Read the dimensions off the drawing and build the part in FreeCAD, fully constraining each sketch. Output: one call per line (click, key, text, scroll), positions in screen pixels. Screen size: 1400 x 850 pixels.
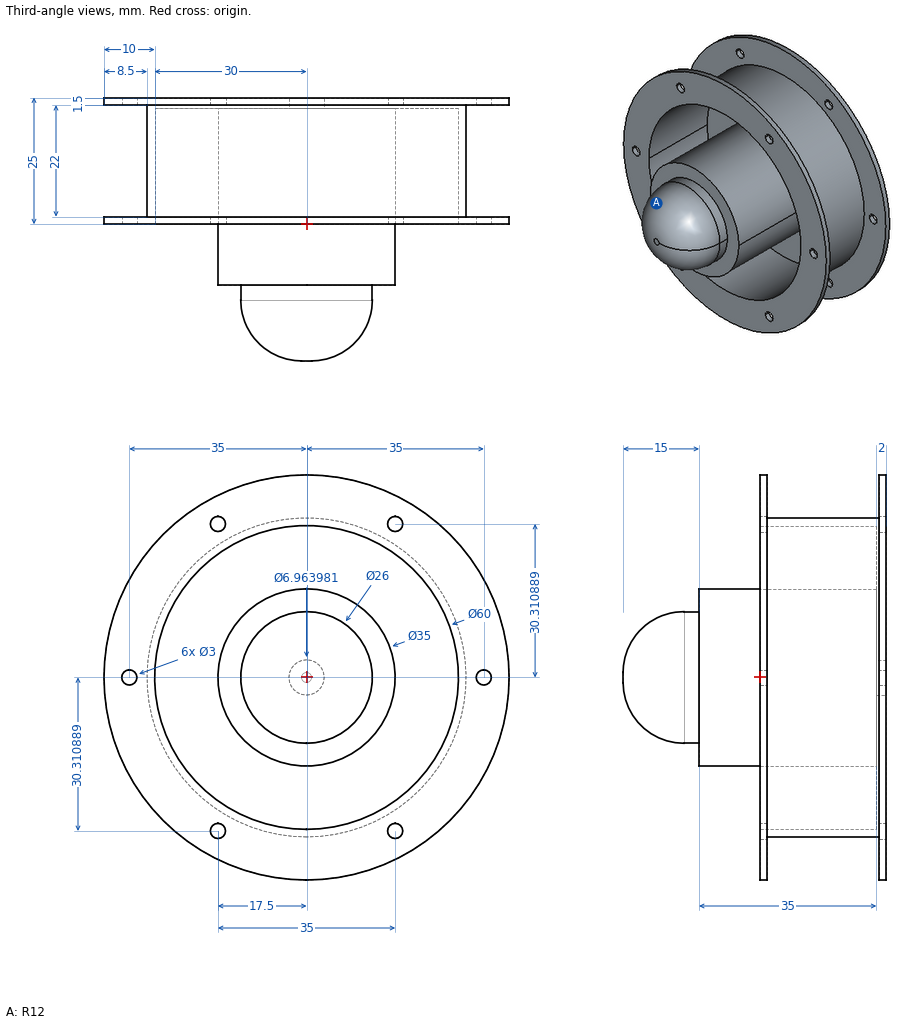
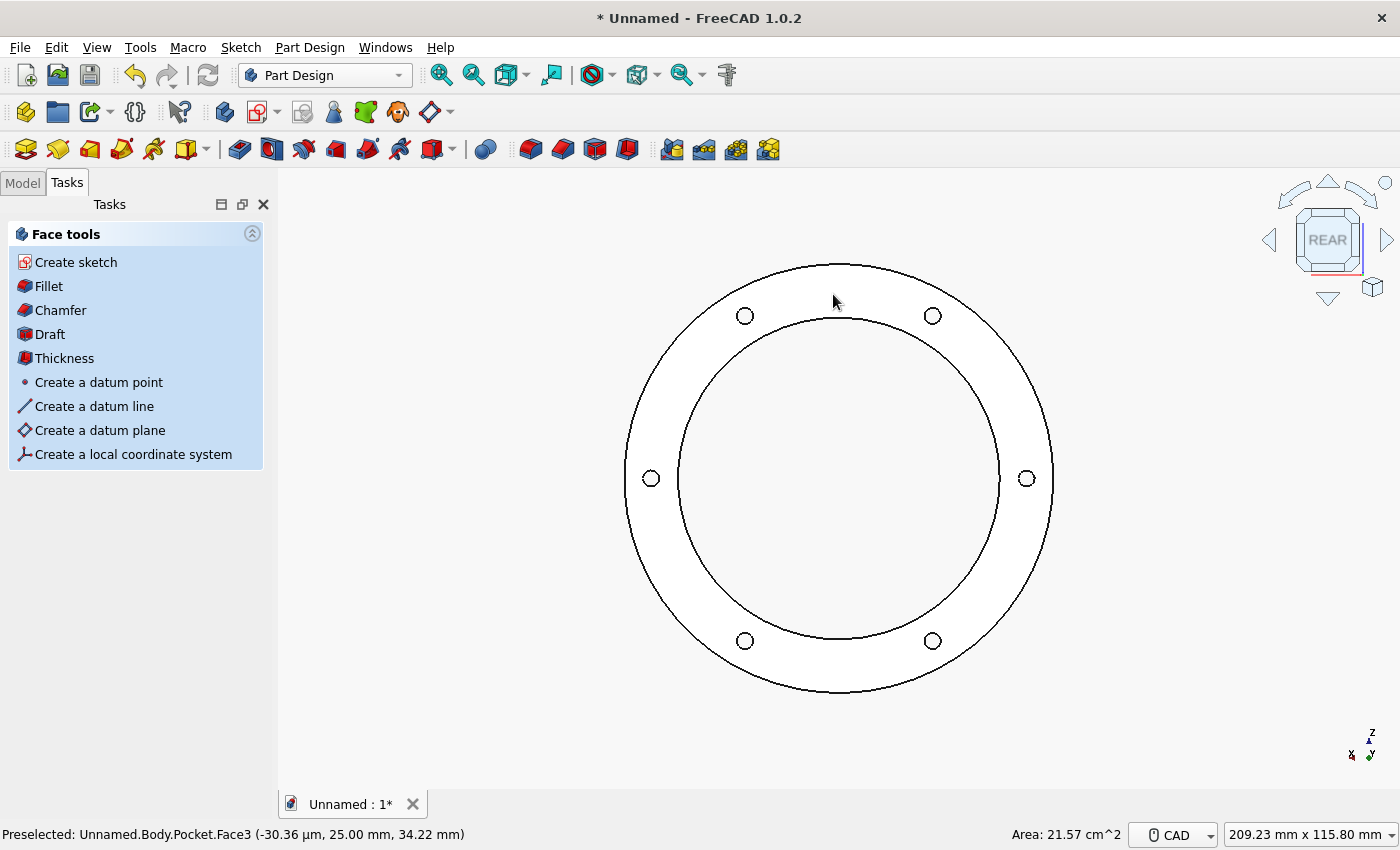
click(258, 112)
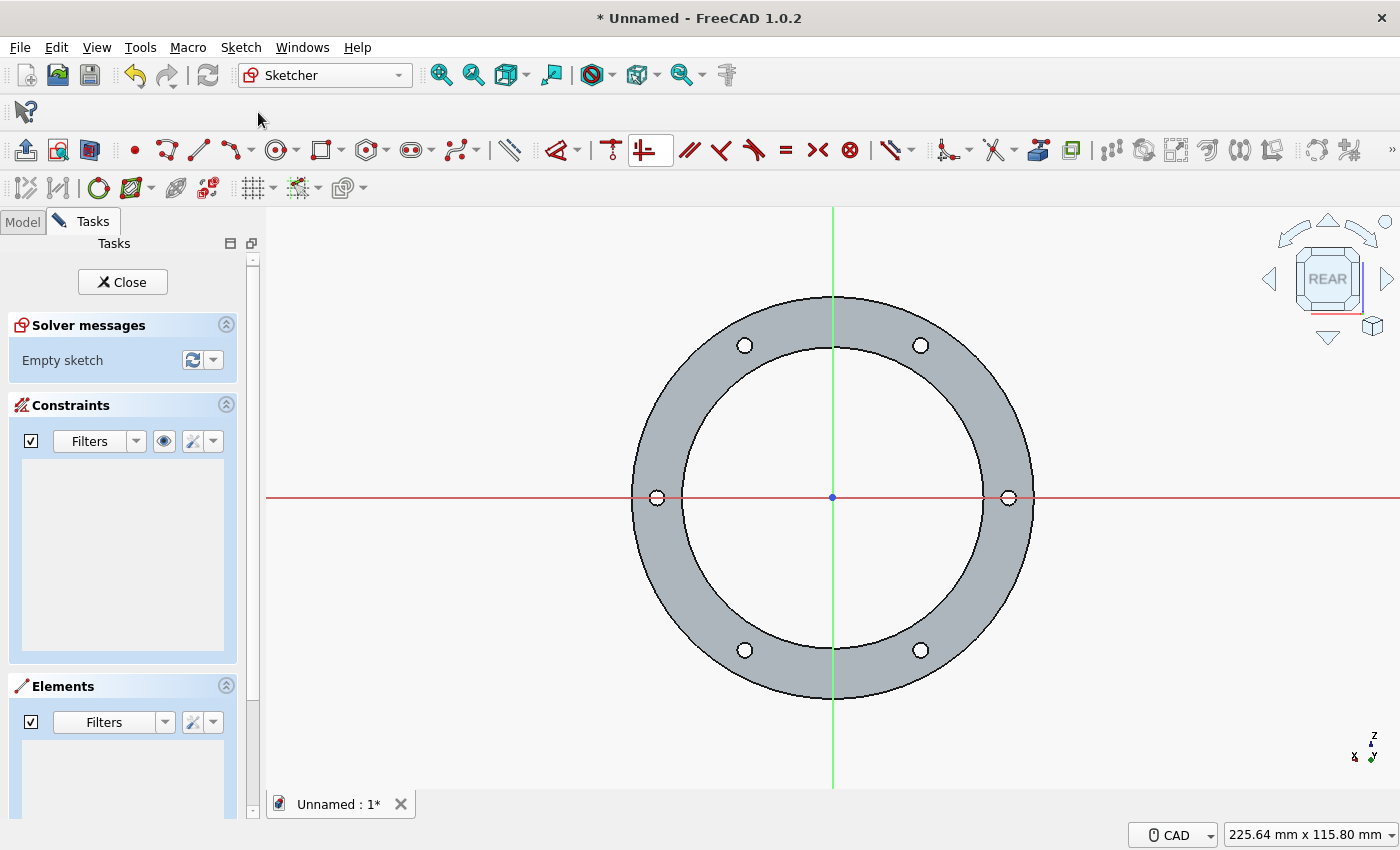
click(276, 150)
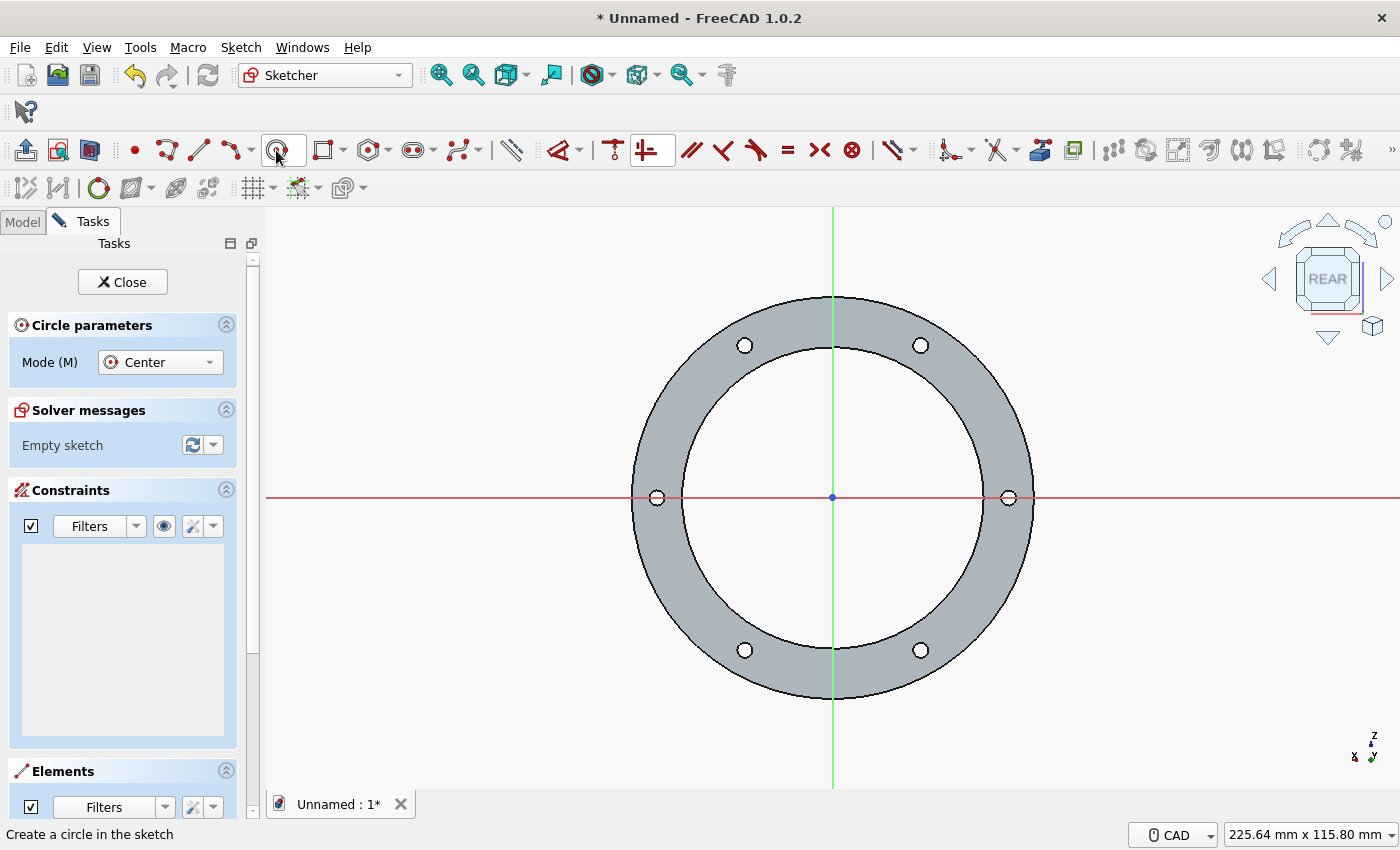
click(833, 498)
click(939, 391)
key(Escape)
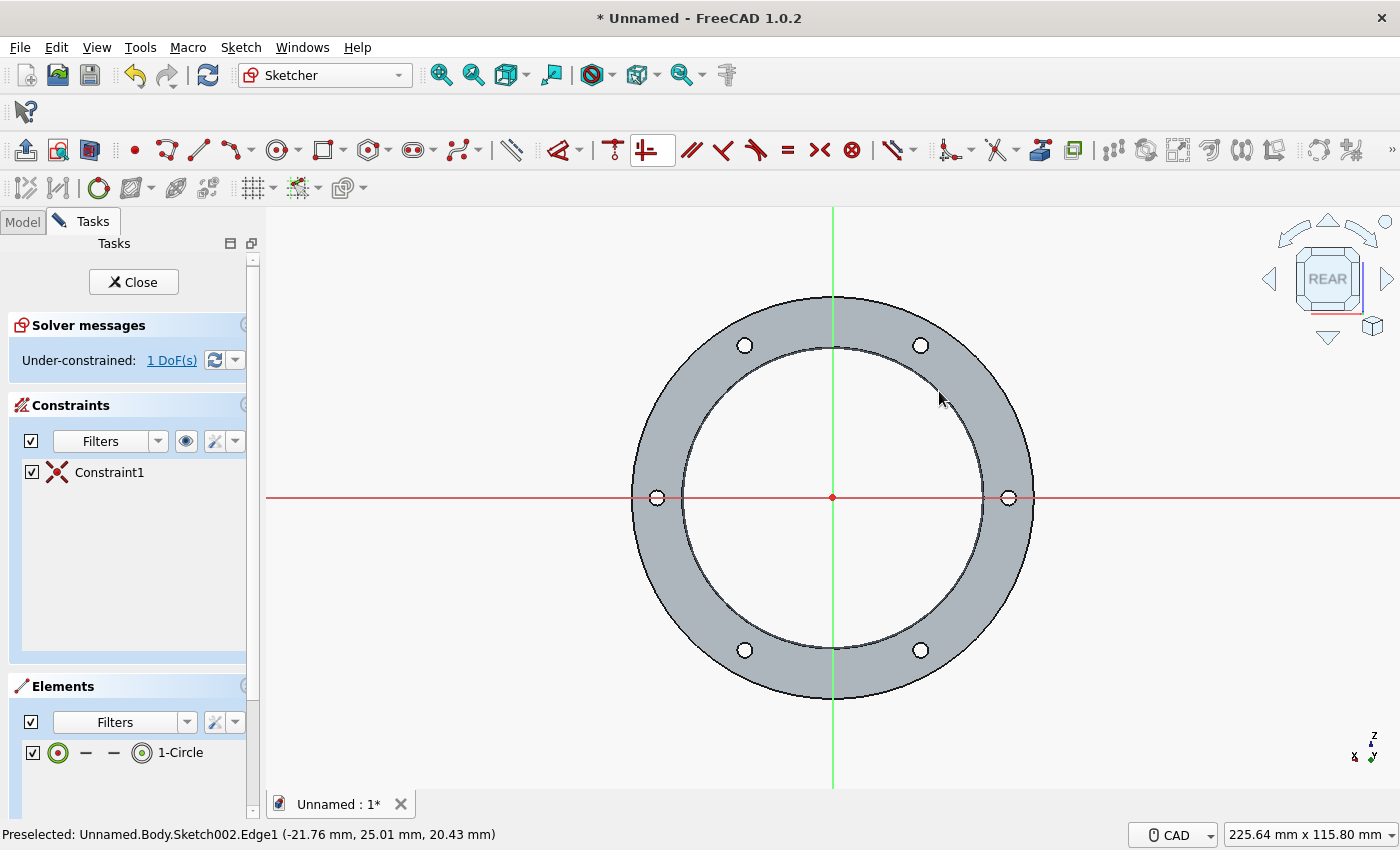
click(558, 150)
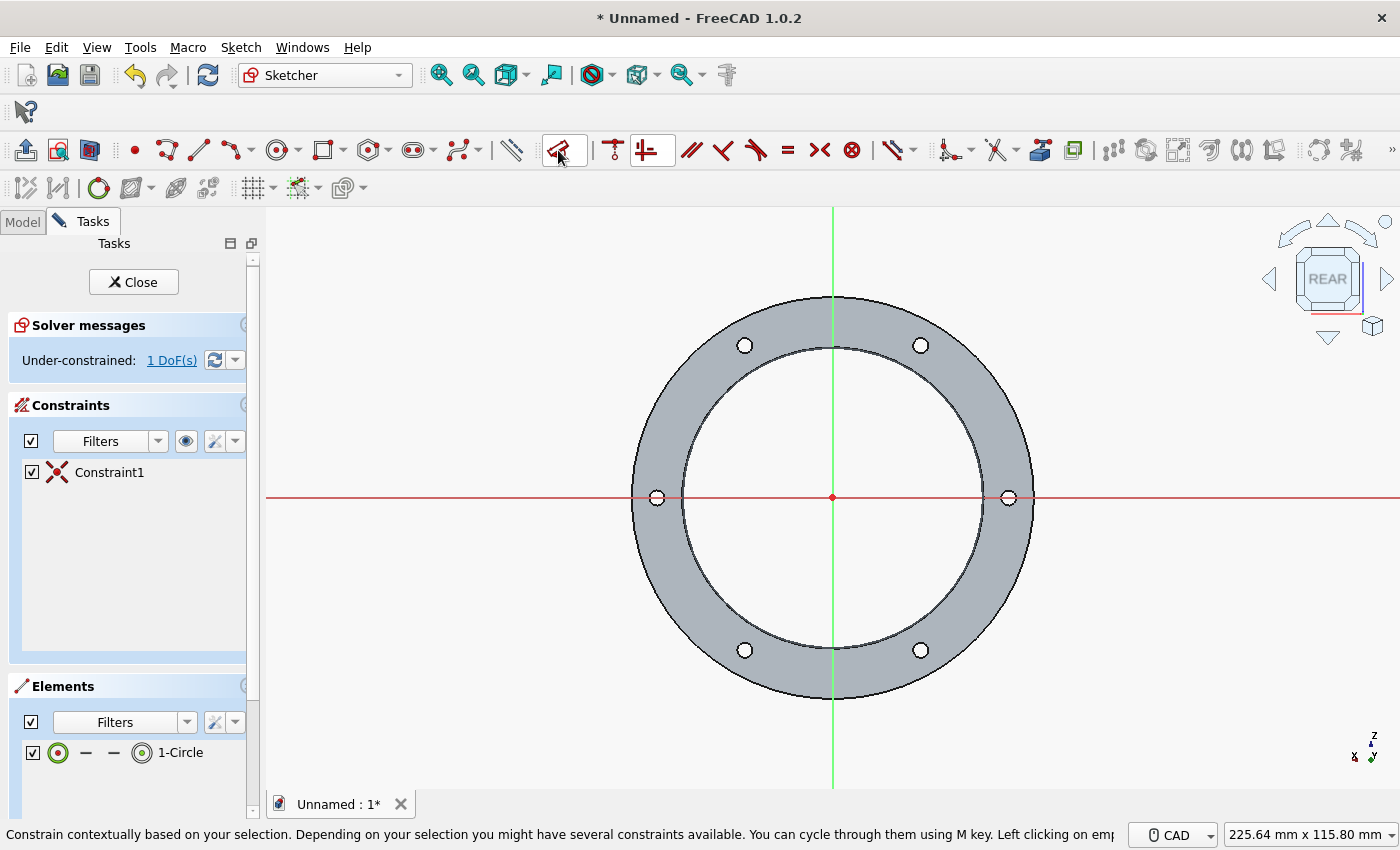
click(939, 392)
click(962, 369)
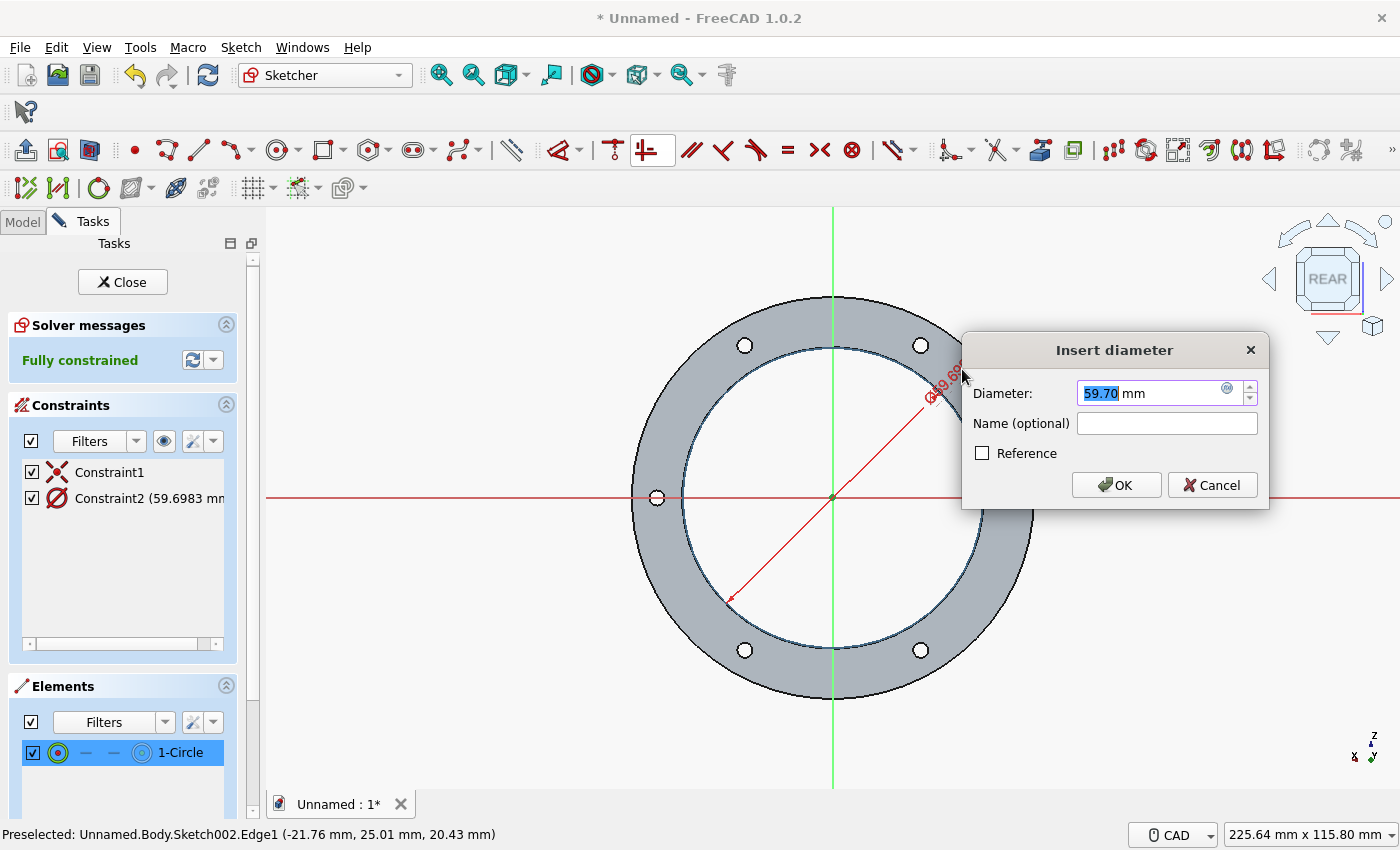
text(60)
key(Return)
key(Escape)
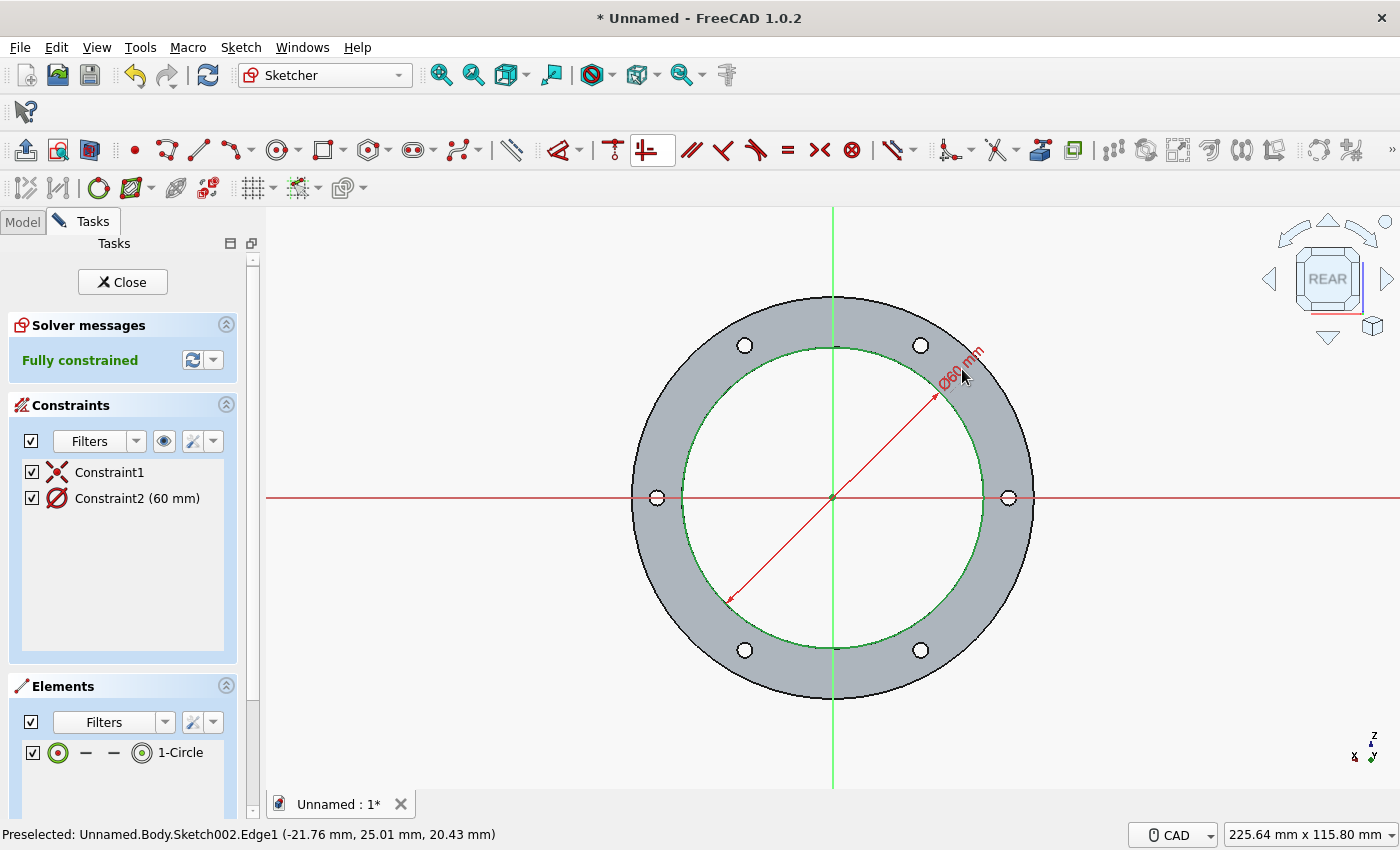
click(123, 282)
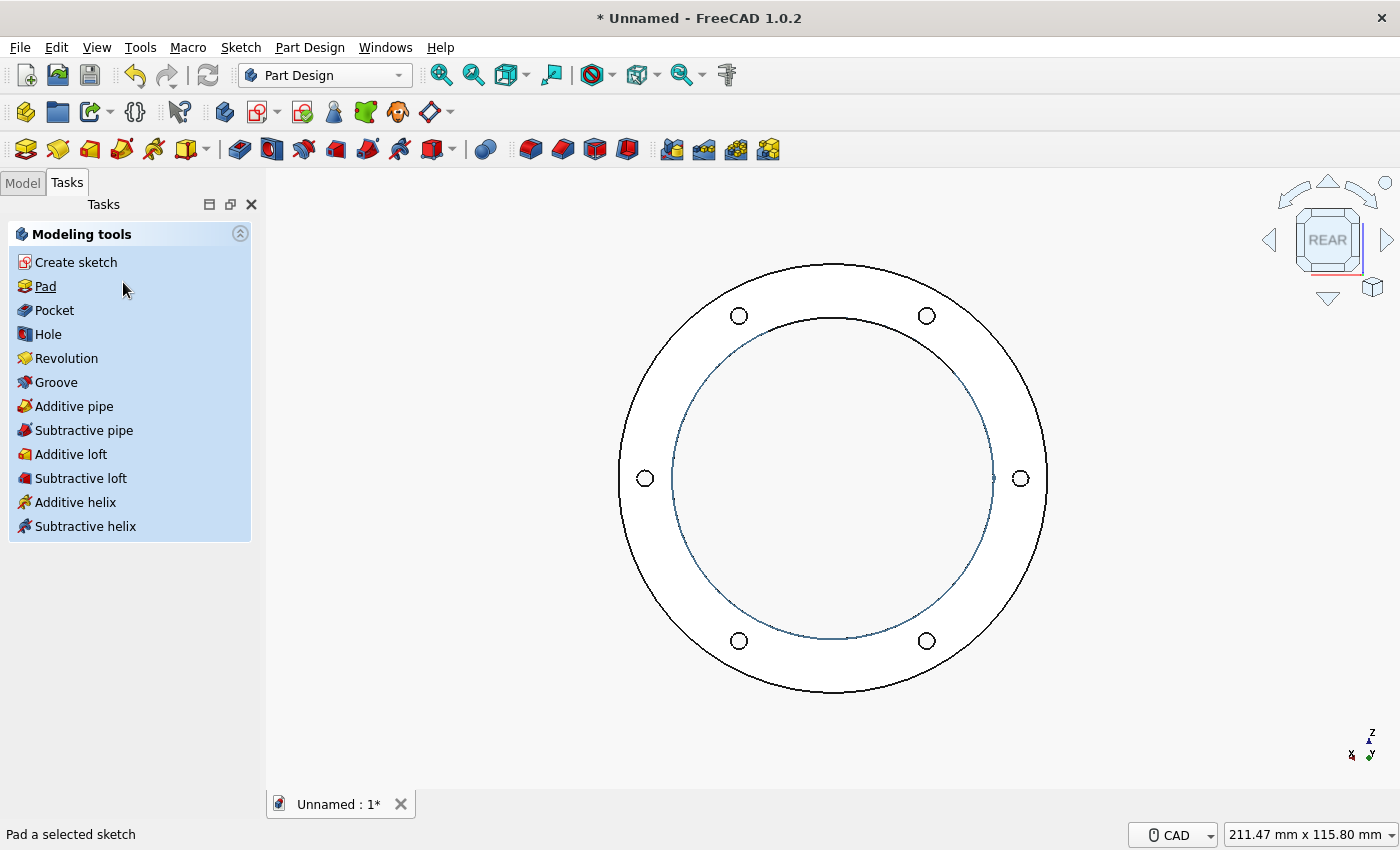
click(26, 150)